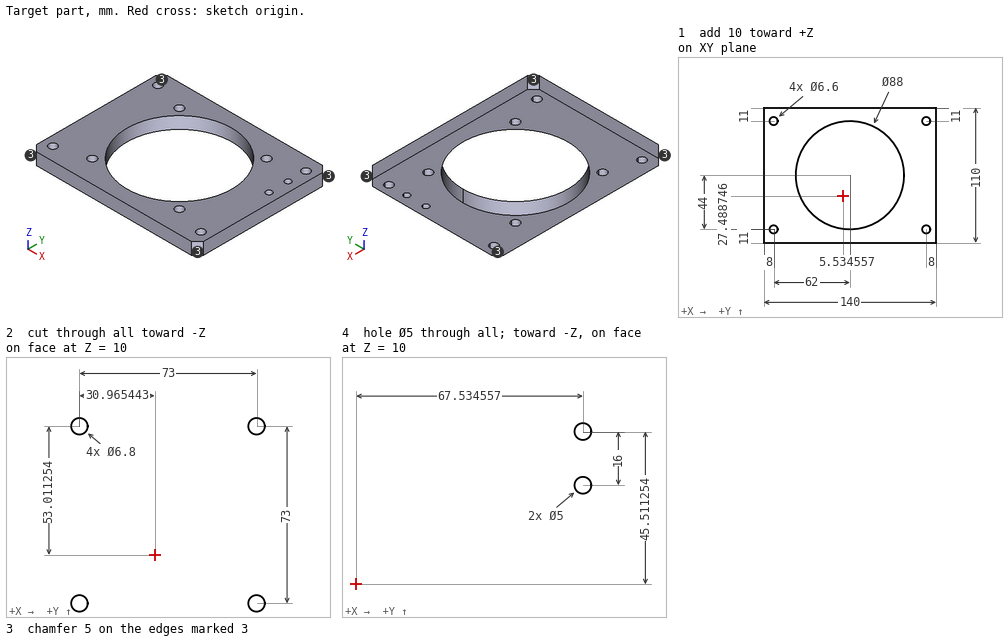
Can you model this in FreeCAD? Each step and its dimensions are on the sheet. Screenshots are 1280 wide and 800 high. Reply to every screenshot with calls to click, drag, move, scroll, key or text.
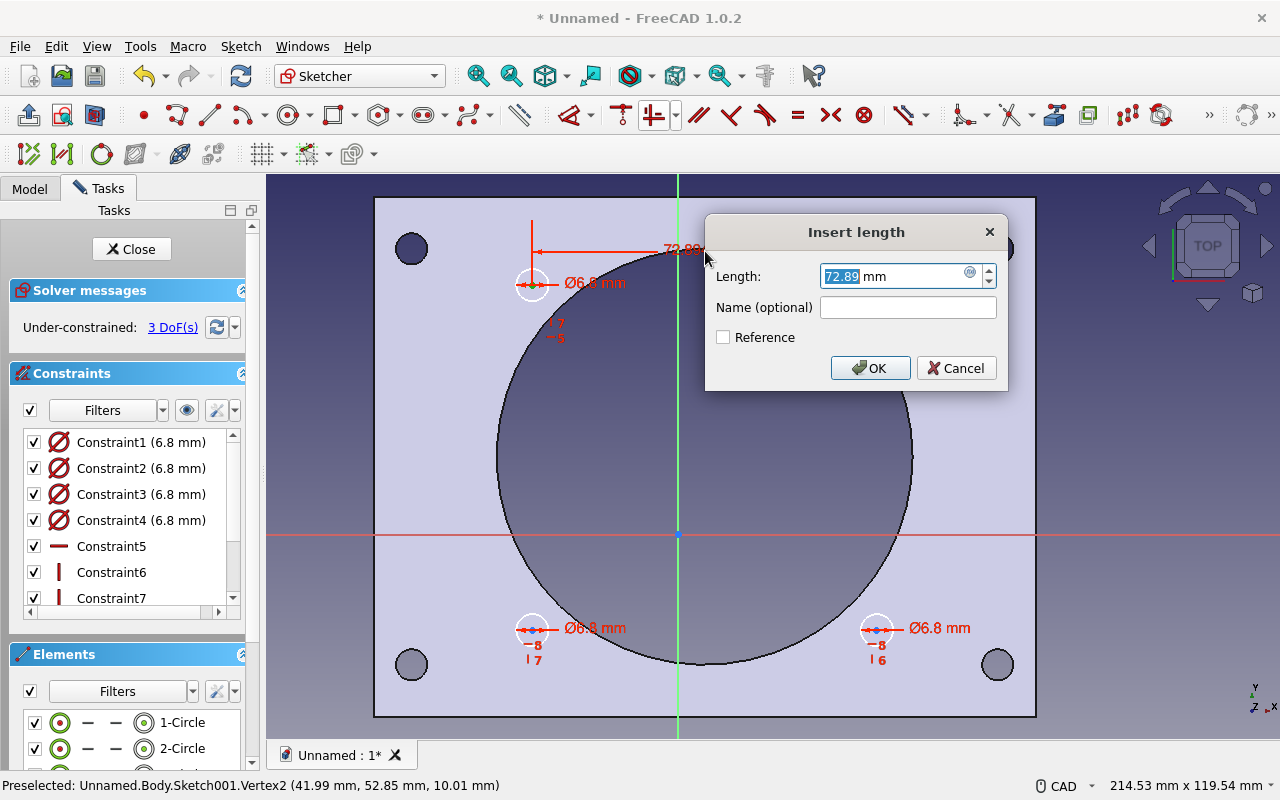
text(73)
key(Return)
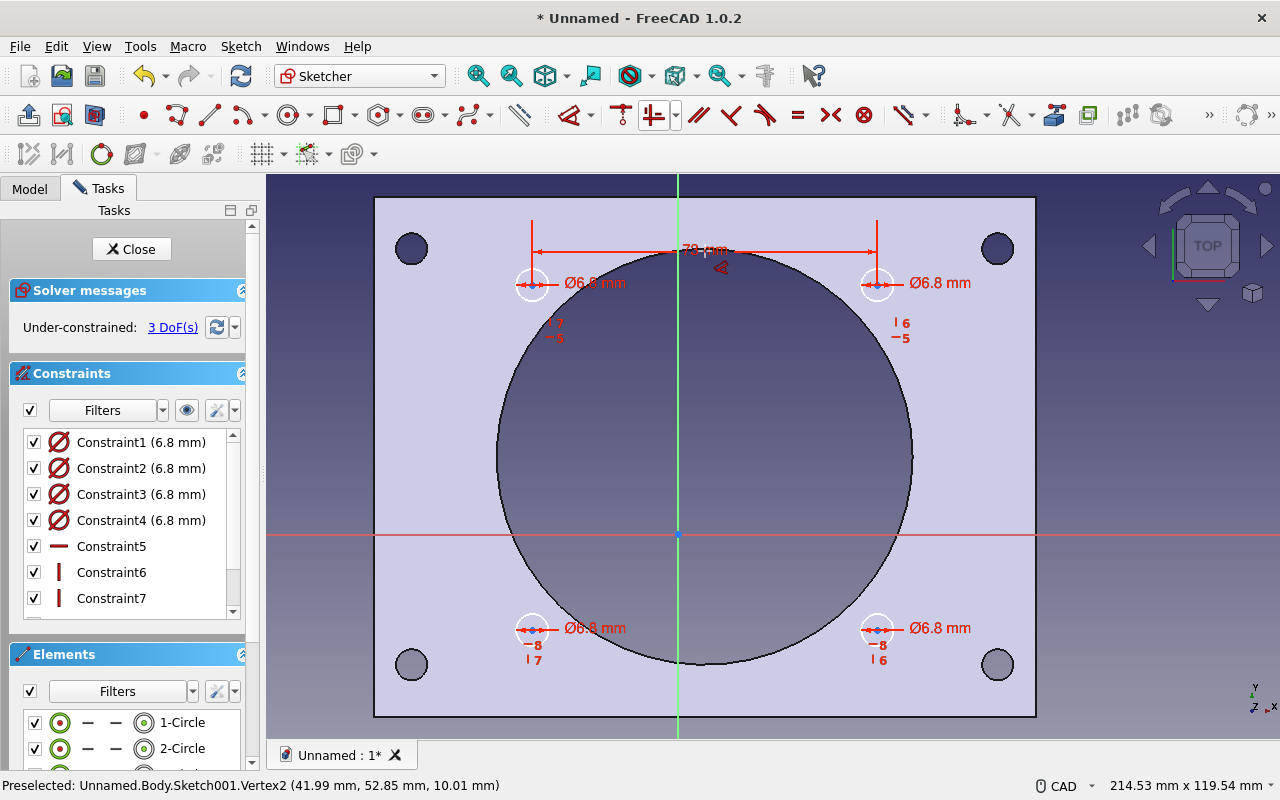
click(877, 285)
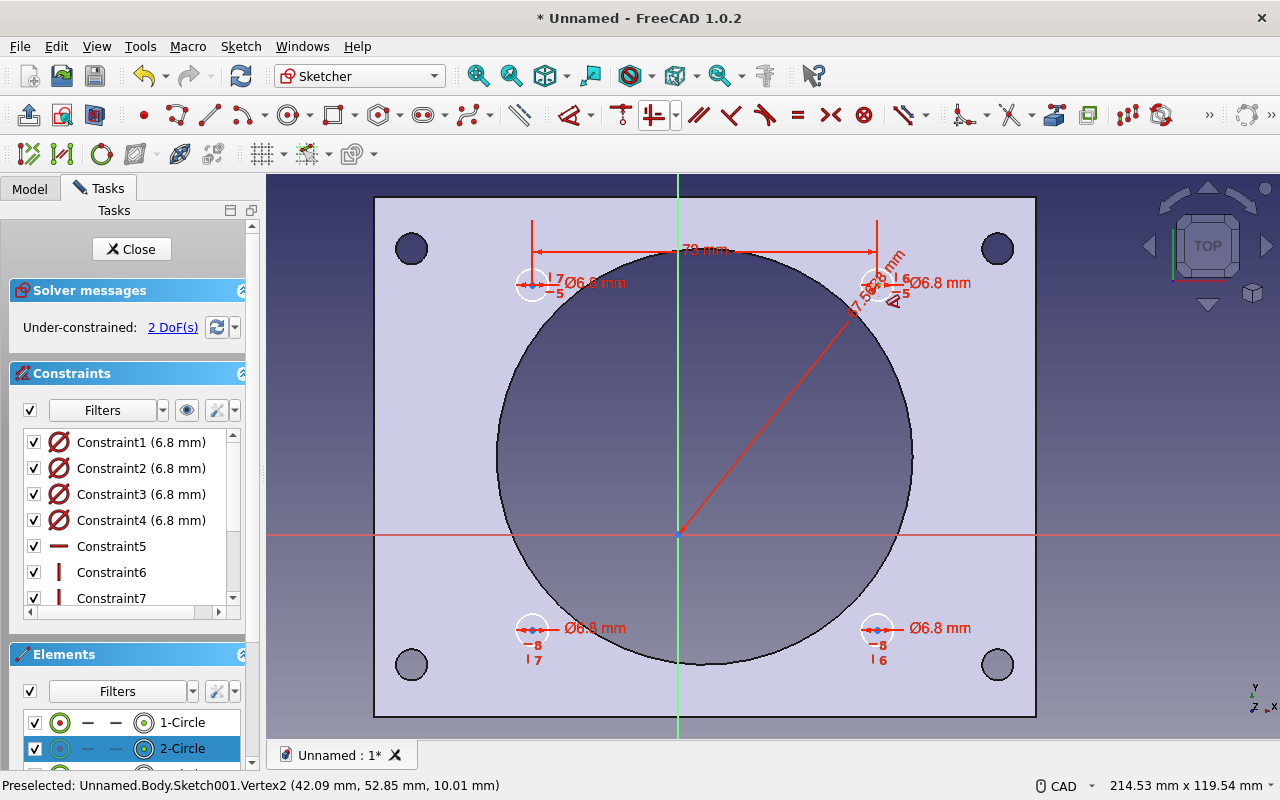
click(877, 630)
click(911, 458)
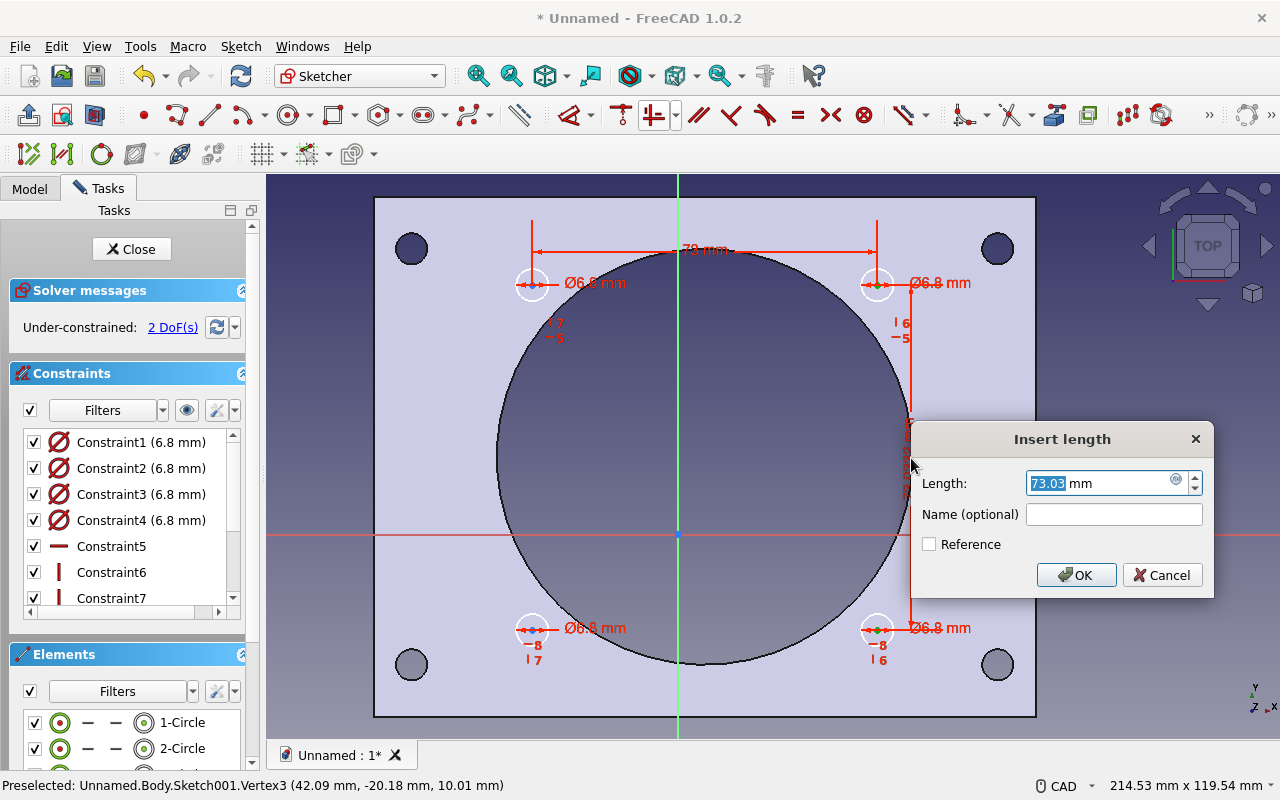
text(73)
key(Return)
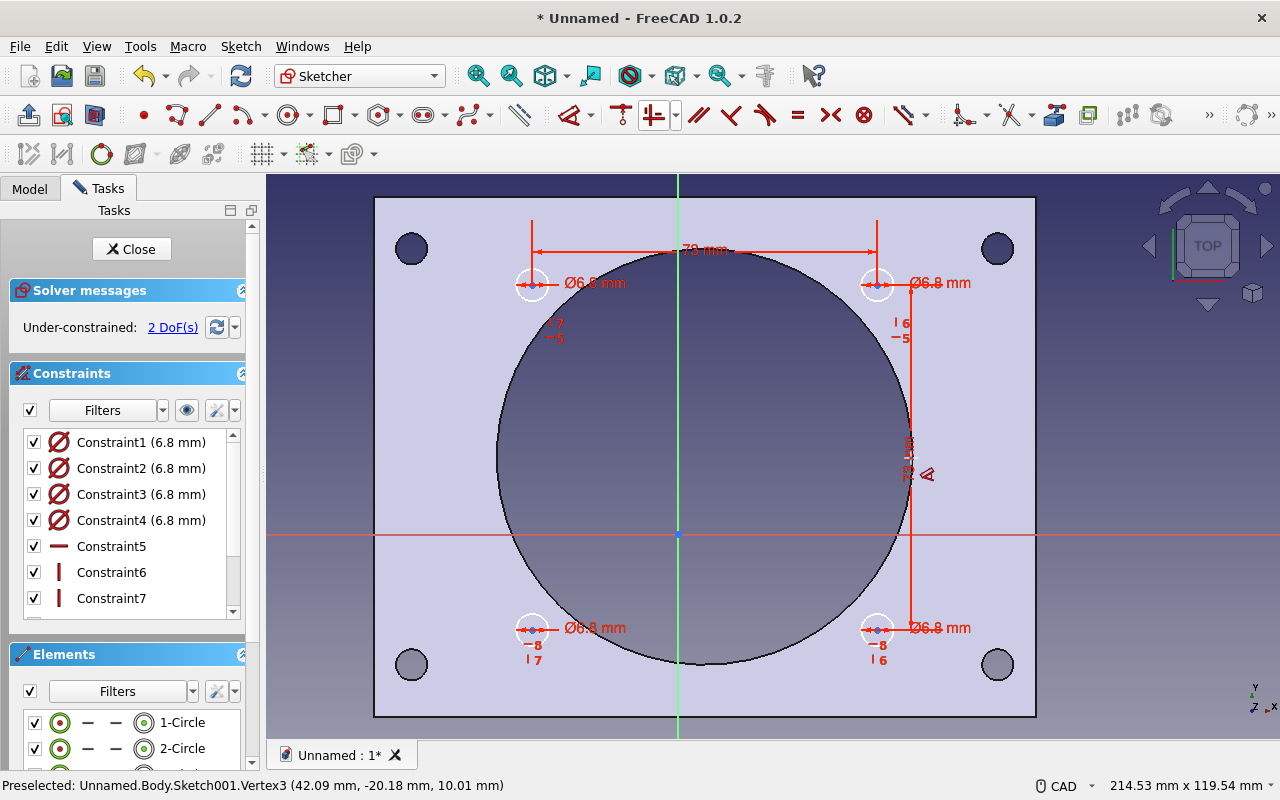
click(532, 285)
click(605, 251)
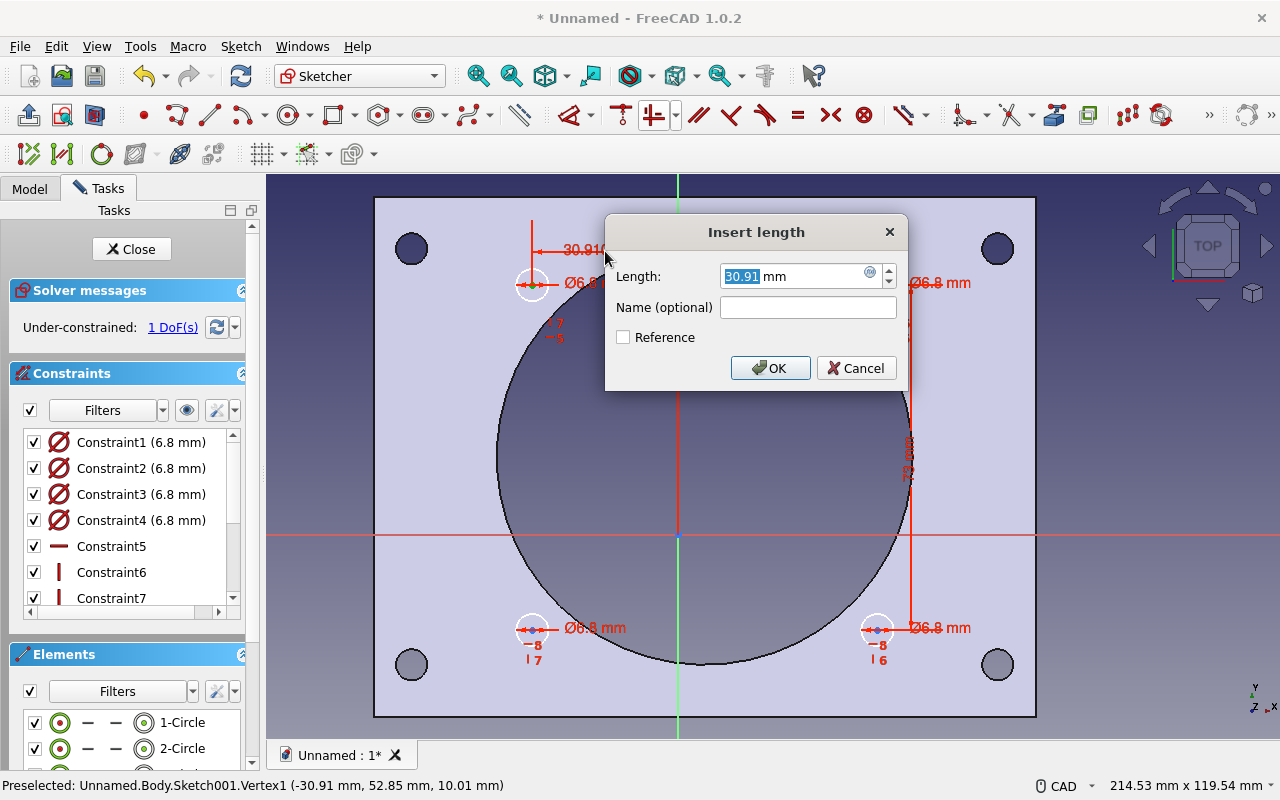
text(30.965443)
key(Return)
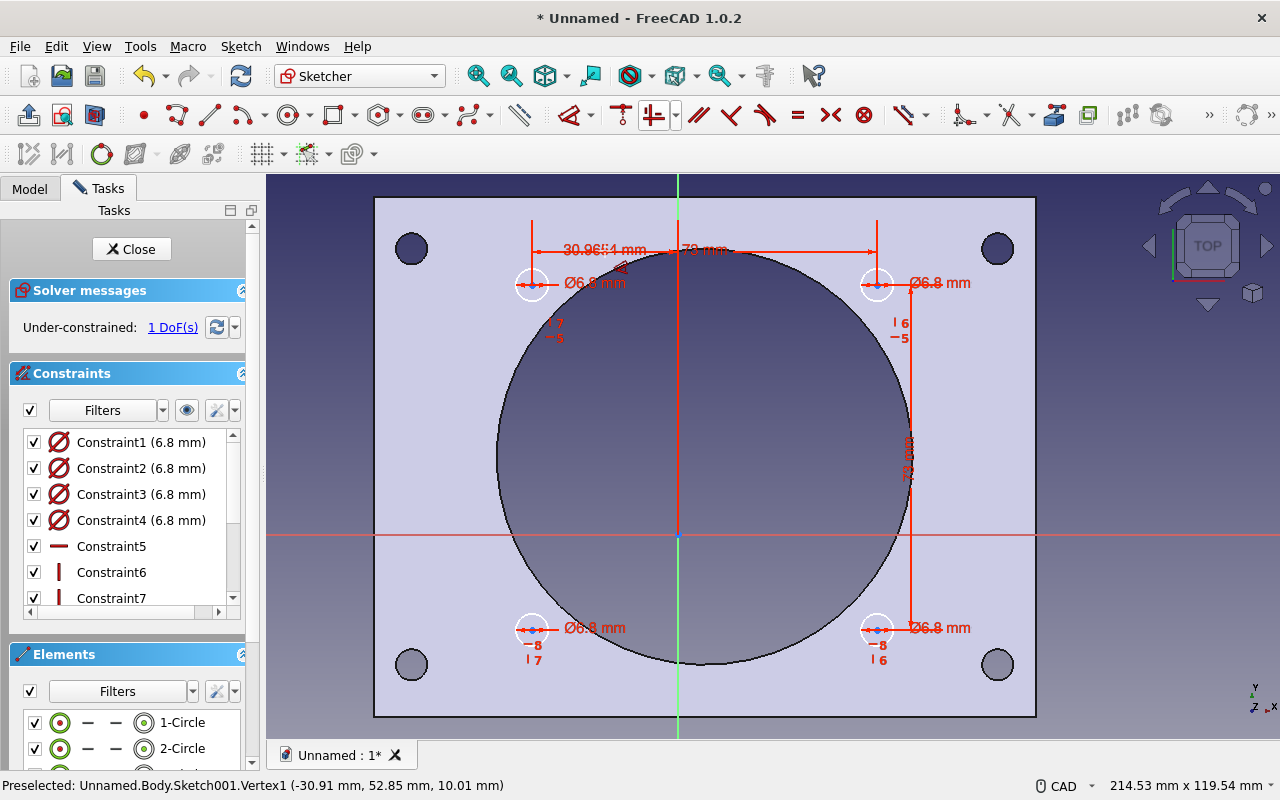
click(532, 285)
click(498, 410)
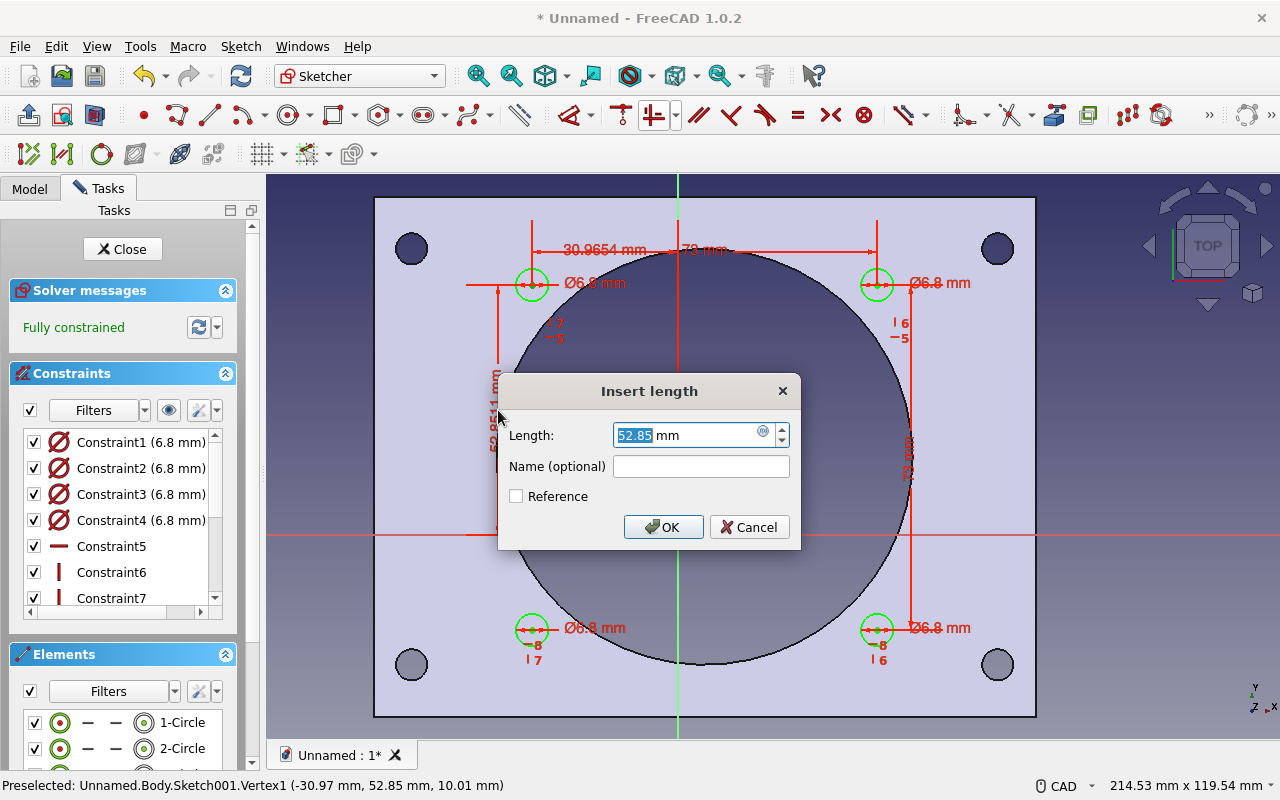
text(53.011254)
key(Return)
key(Escape)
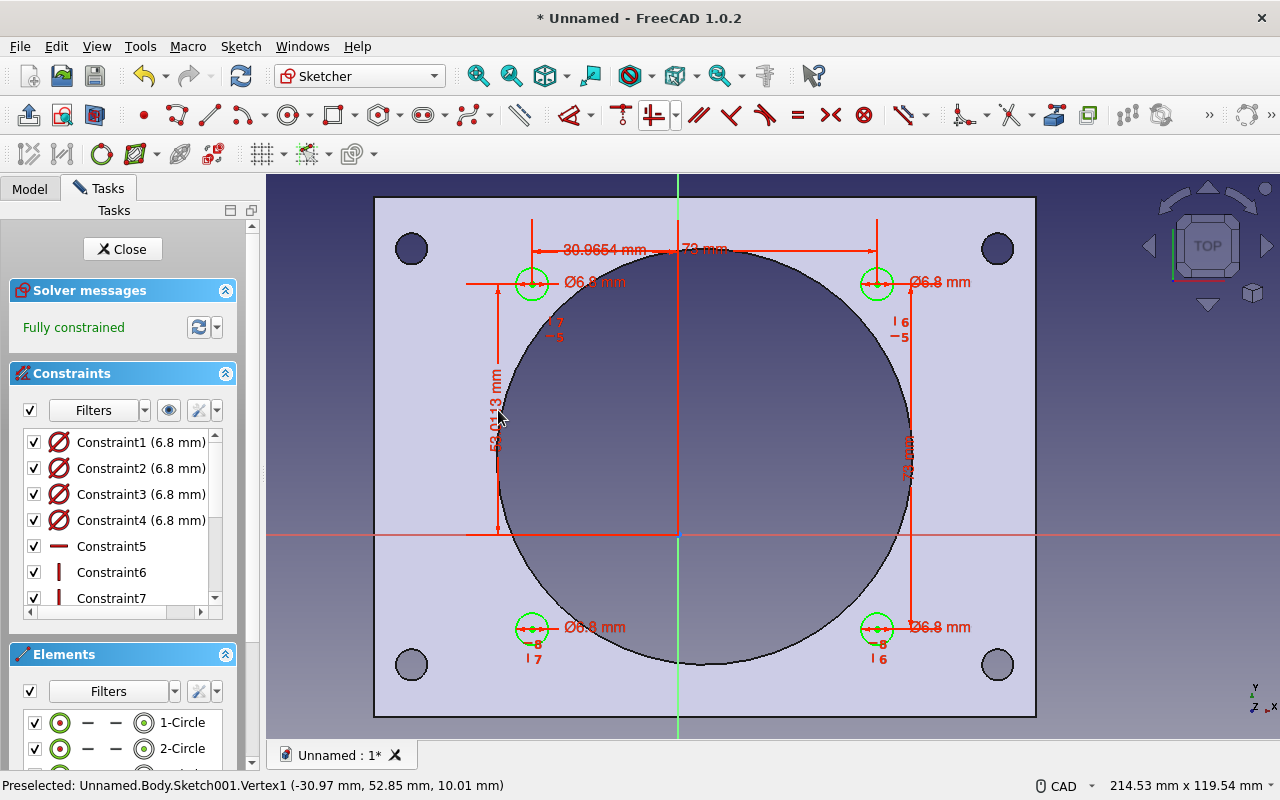
click(123, 249)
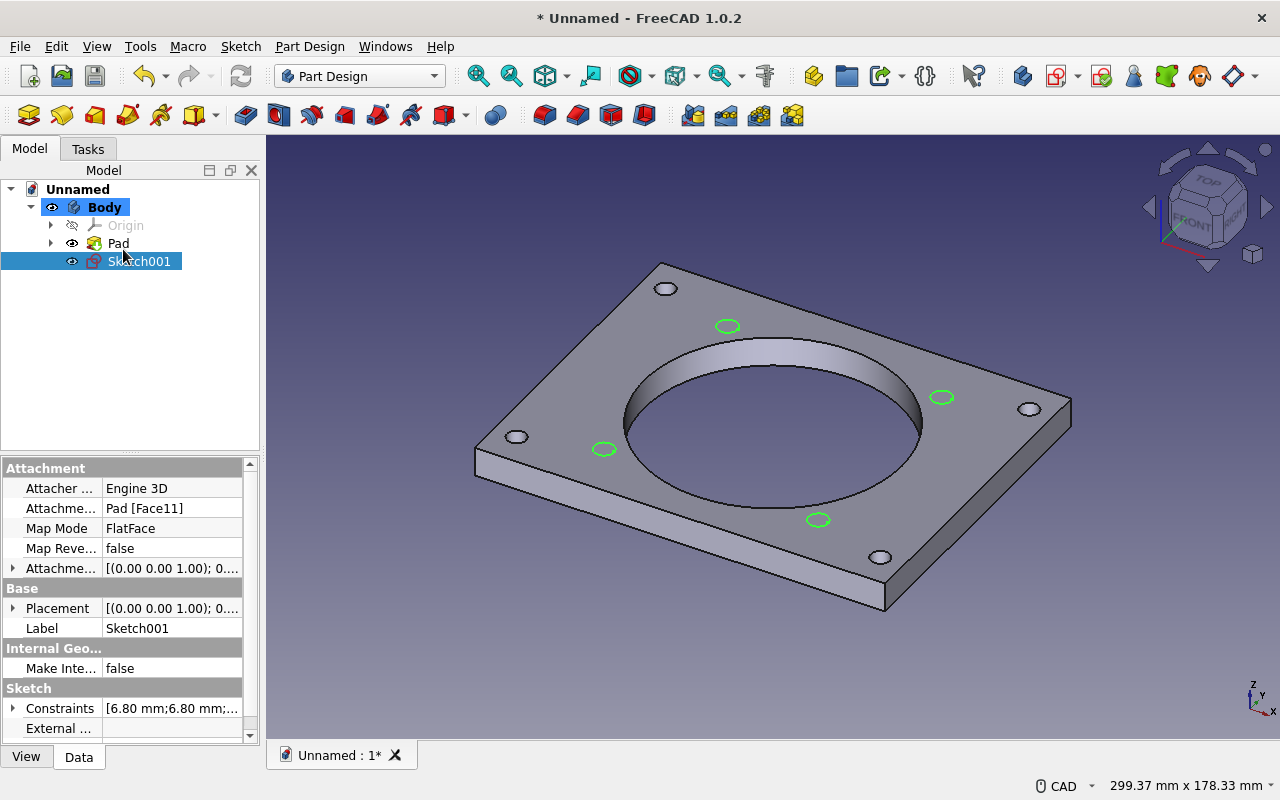
click(246, 116)